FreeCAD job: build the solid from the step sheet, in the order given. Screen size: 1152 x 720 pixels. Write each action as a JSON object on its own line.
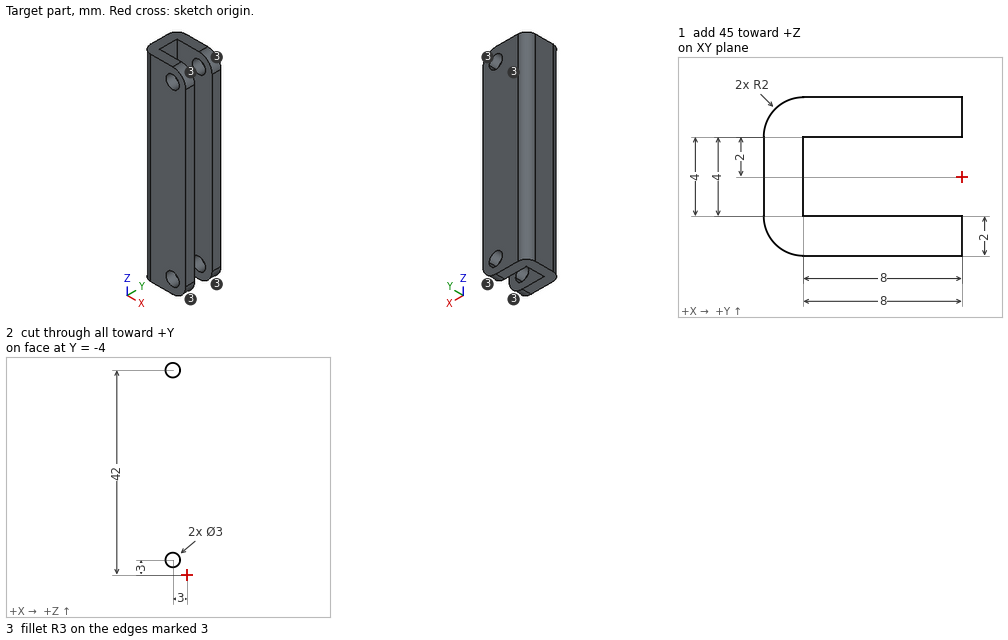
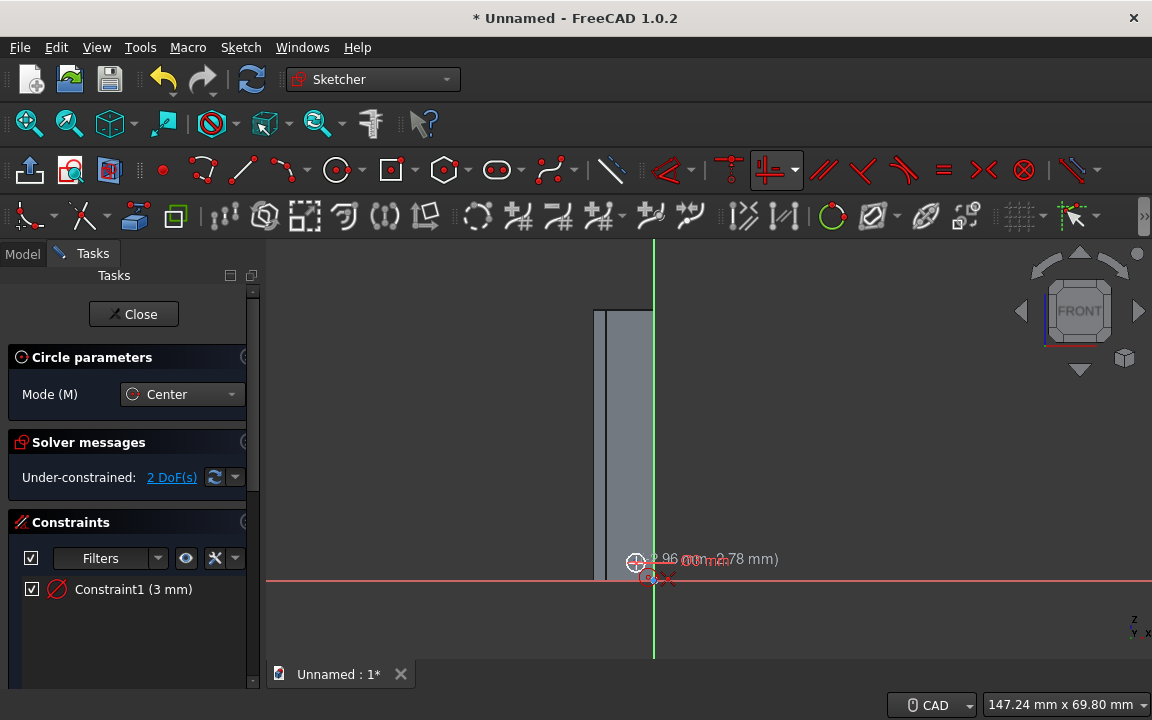
{"action": "scroll", "coordinate": [636, 328], "scroll_direction": "up", "scroll_amount": 5}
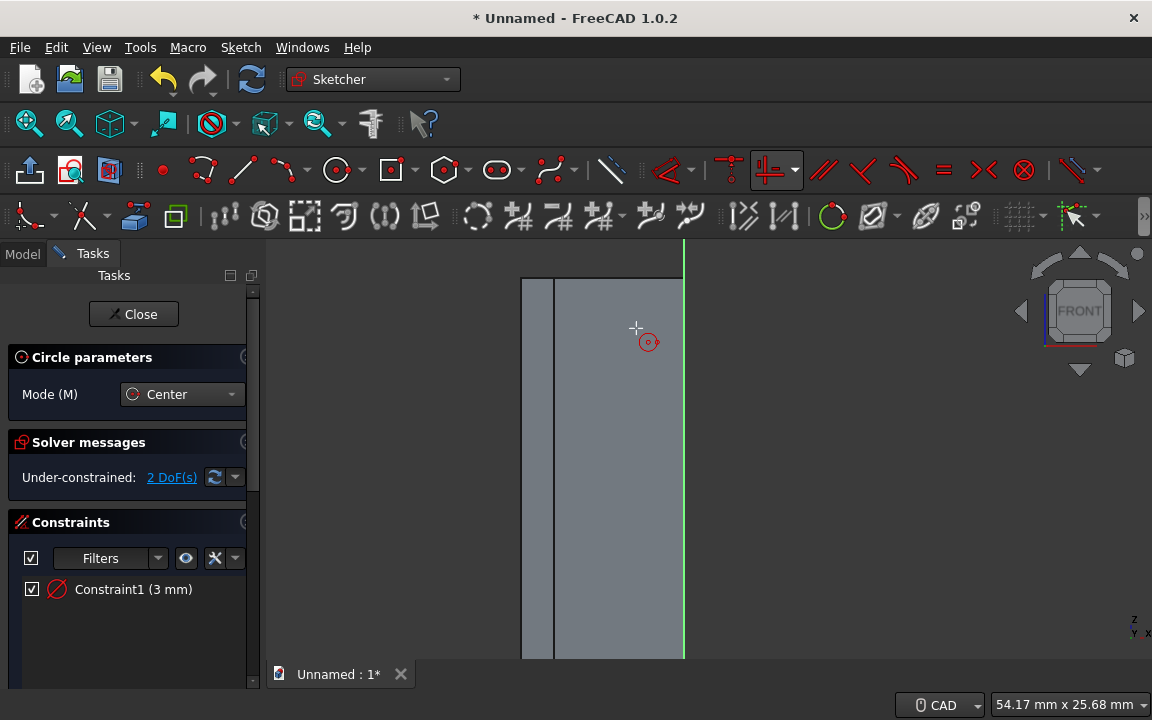
{"action": "left_click", "coordinate": [635, 327]}
{"action": "mouse_move", "coordinate": [653, 310]}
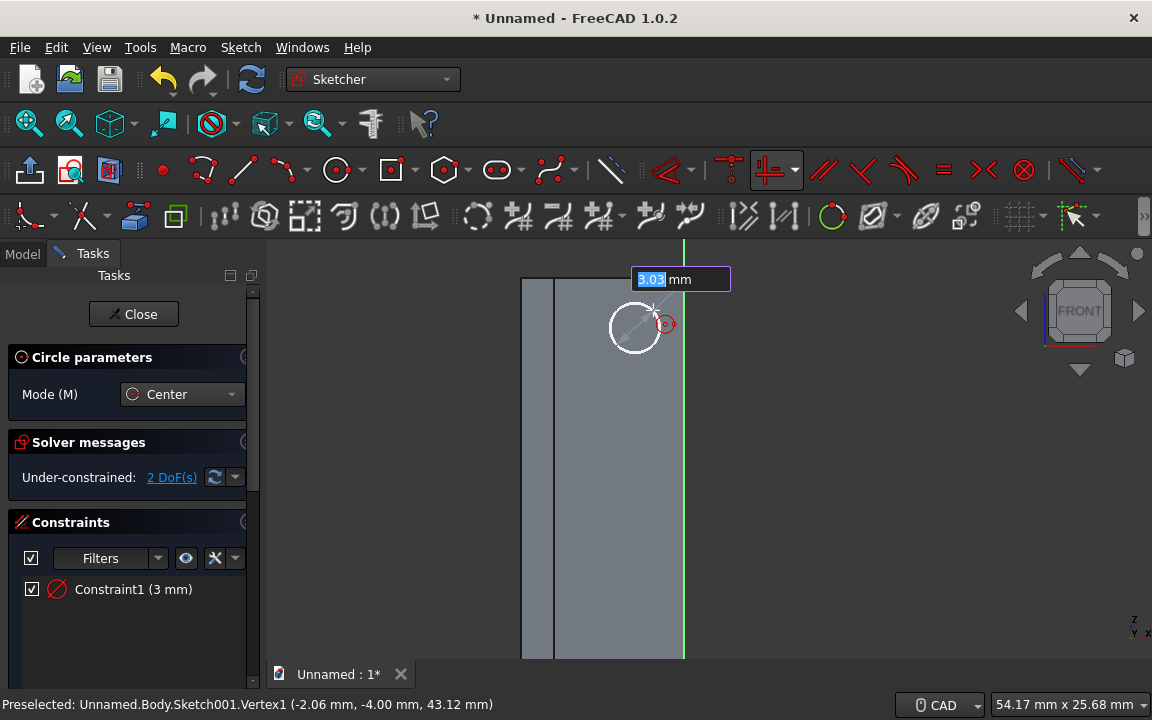
{"action": "type", "text": "3"}
{"action": "key", "text": "Return"}
{"action": "key", "text": "Escape"}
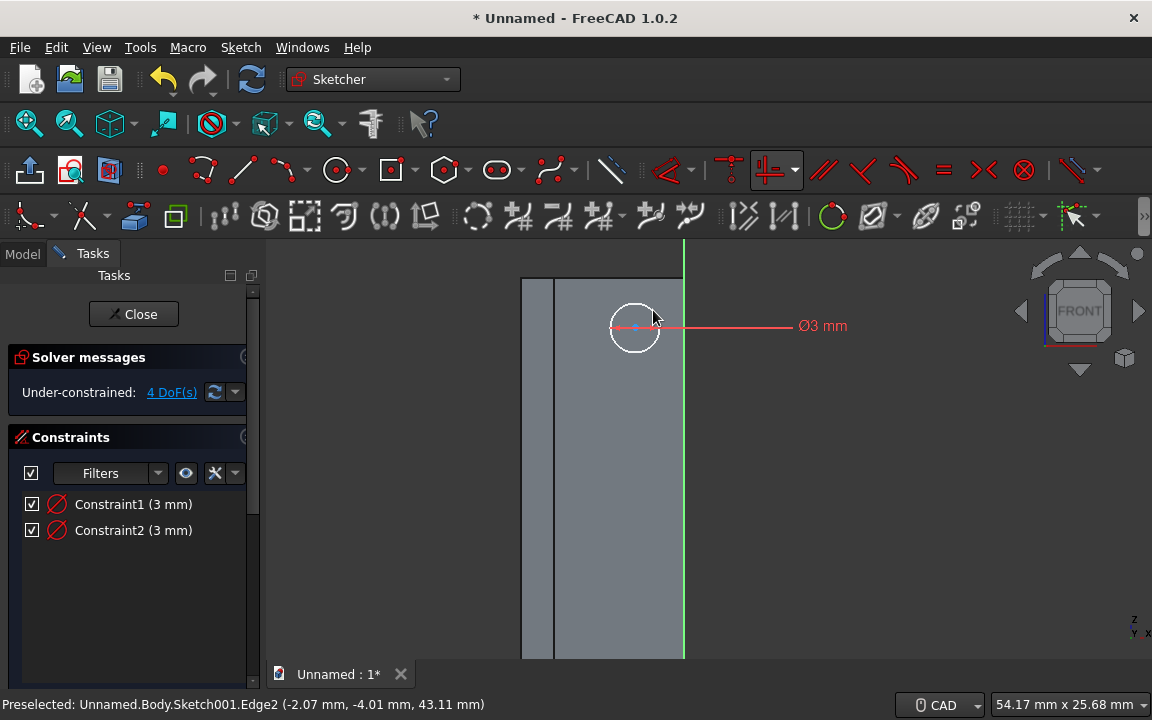
{"action": "scroll", "coordinate": [636, 327], "scroll_direction": "down", "scroll_amount": 5}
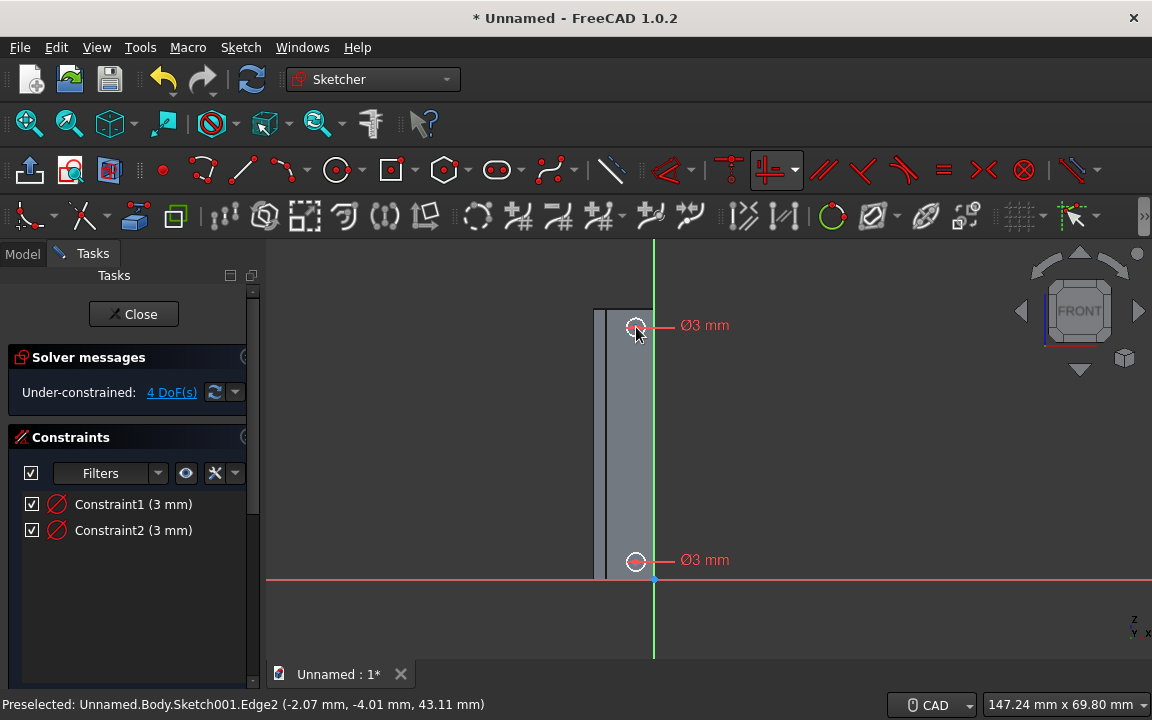
{"action": "left_click", "coordinate": [636, 562]}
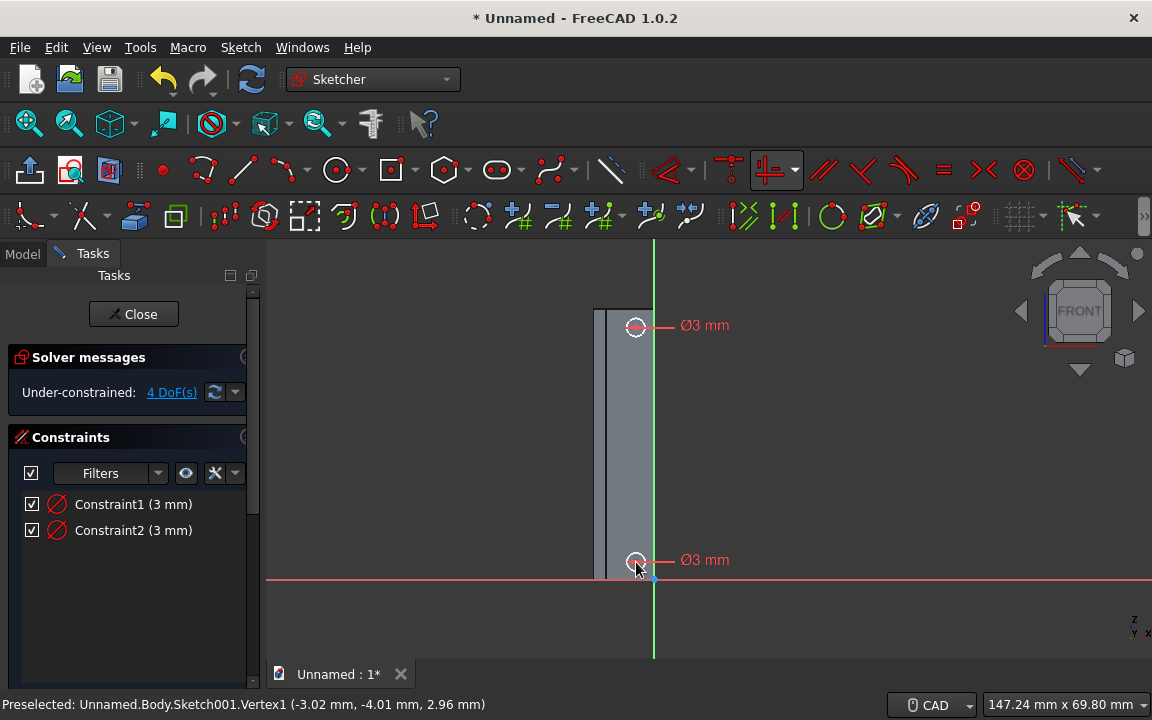
{"action": "left_click", "coordinate": [636, 328]}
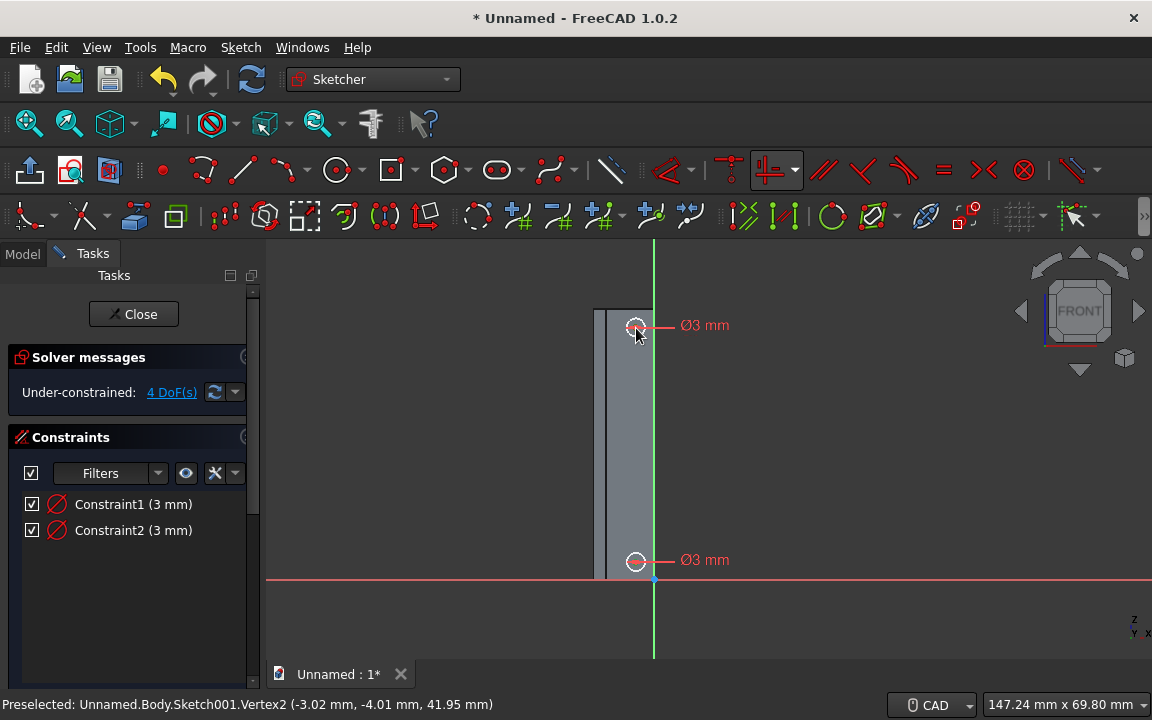
{"action": "left_click", "coordinate": [798, 170]}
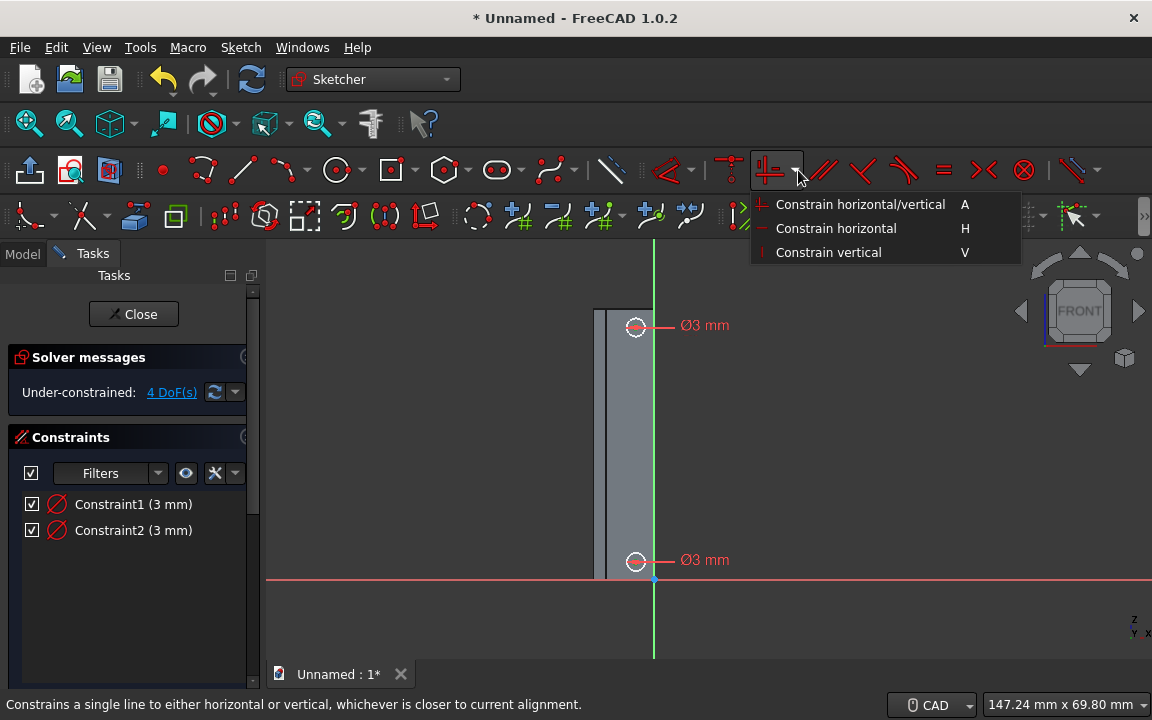
{"action": "left_click", "coordinate": [886, 252]}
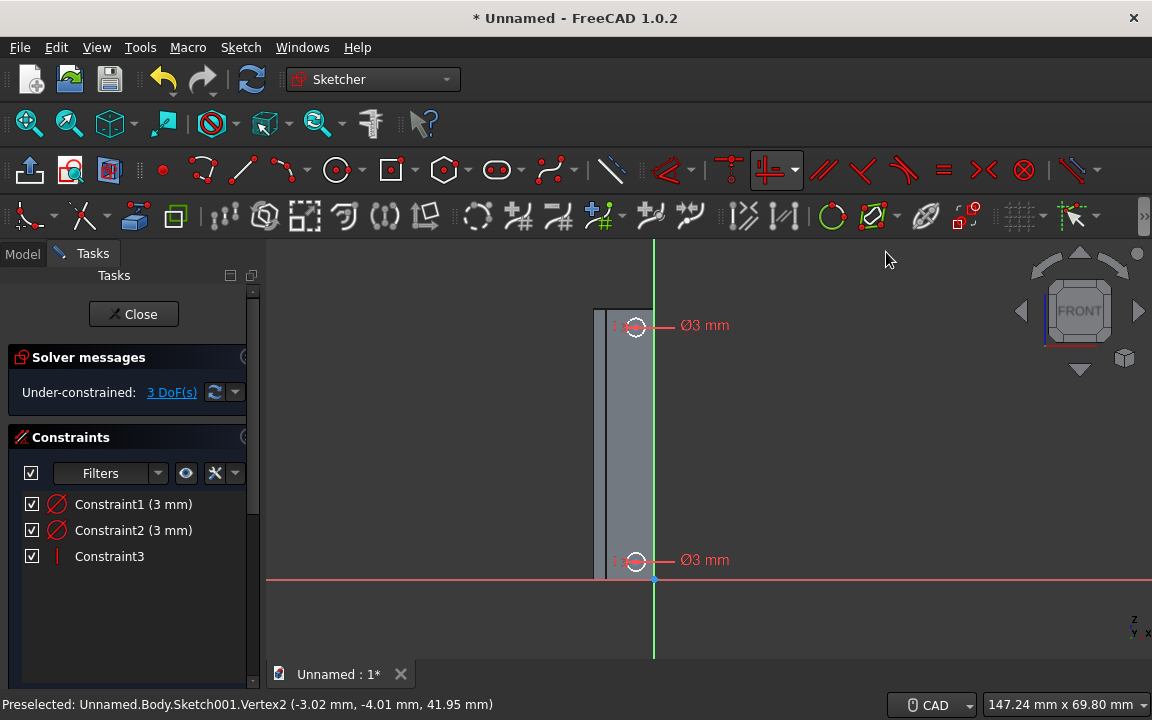
{"action": "left_click", "coordinate": [666, 170]}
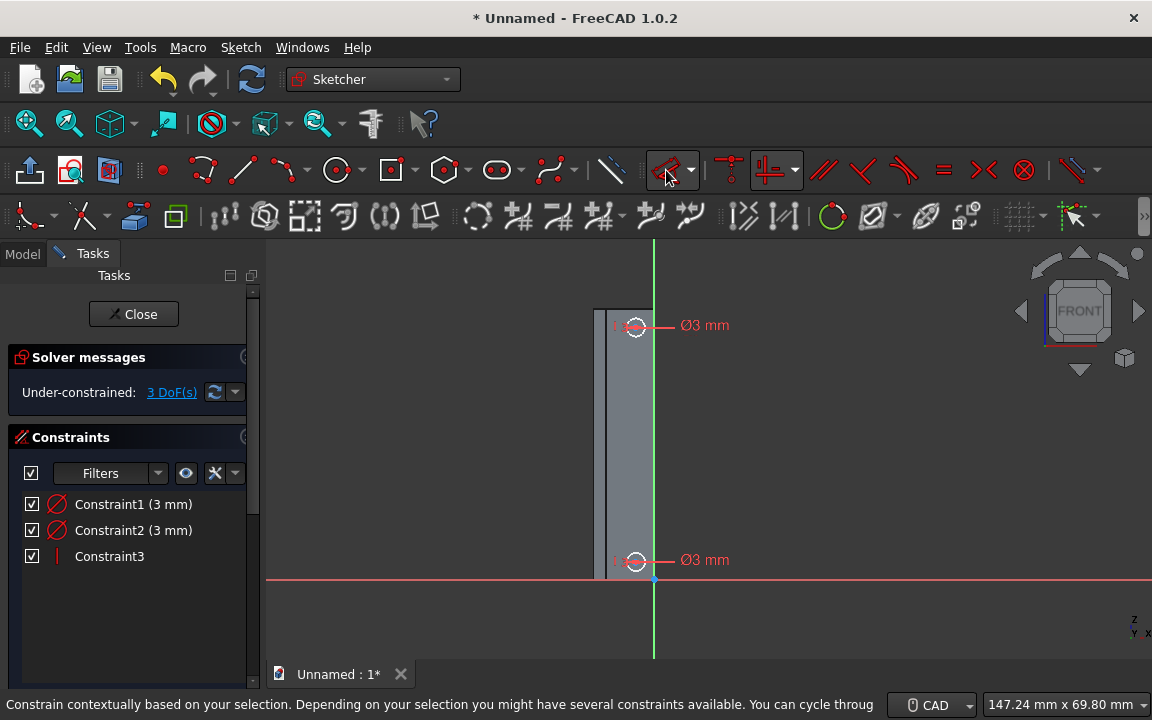
{"action": "scroll", "coordinate": [636, 562], "scroll_direction": "up", "scroll_amount": 4}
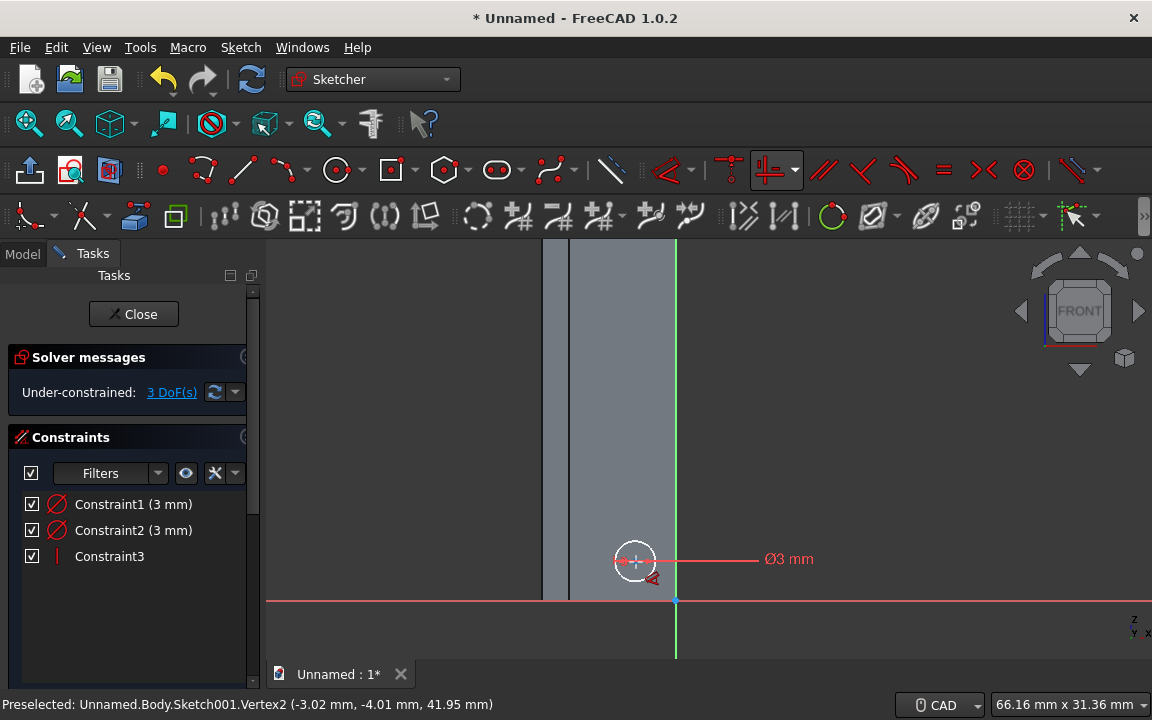
{"action": "left_click", "coordinate": [635, 561]}
{"action": "left_click", "coordinate": [656, 527]}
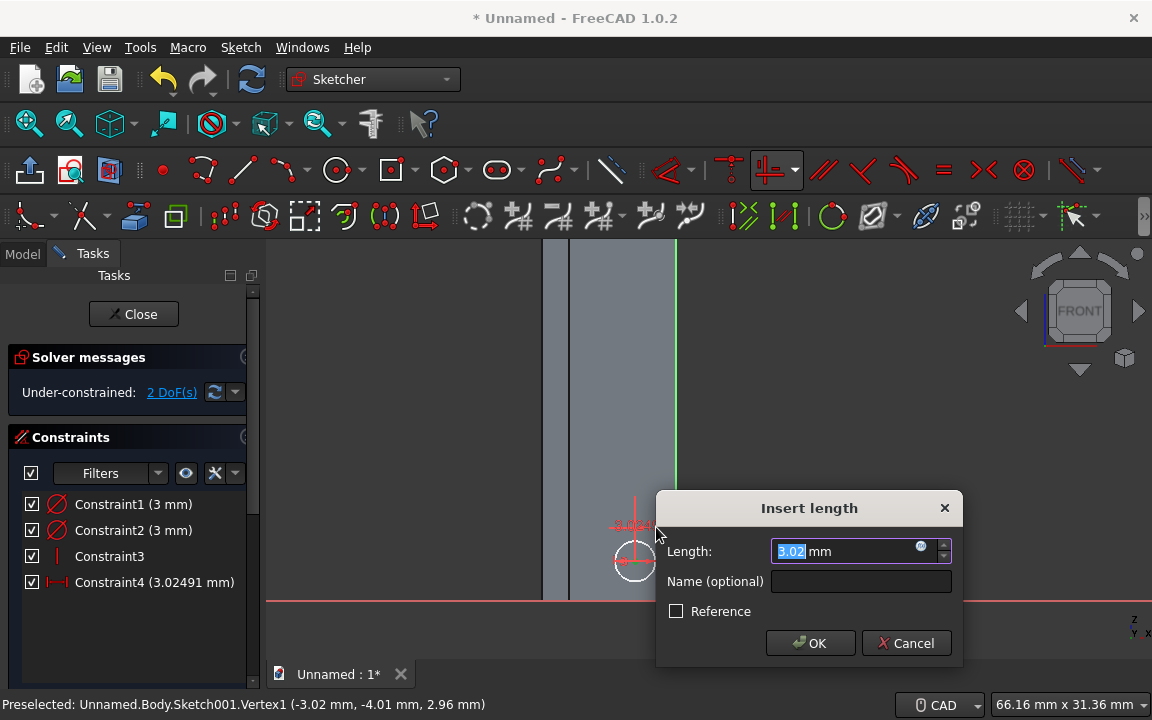
{"action": "type", "text": "3"}
{"action": "key", "text": "Return"}